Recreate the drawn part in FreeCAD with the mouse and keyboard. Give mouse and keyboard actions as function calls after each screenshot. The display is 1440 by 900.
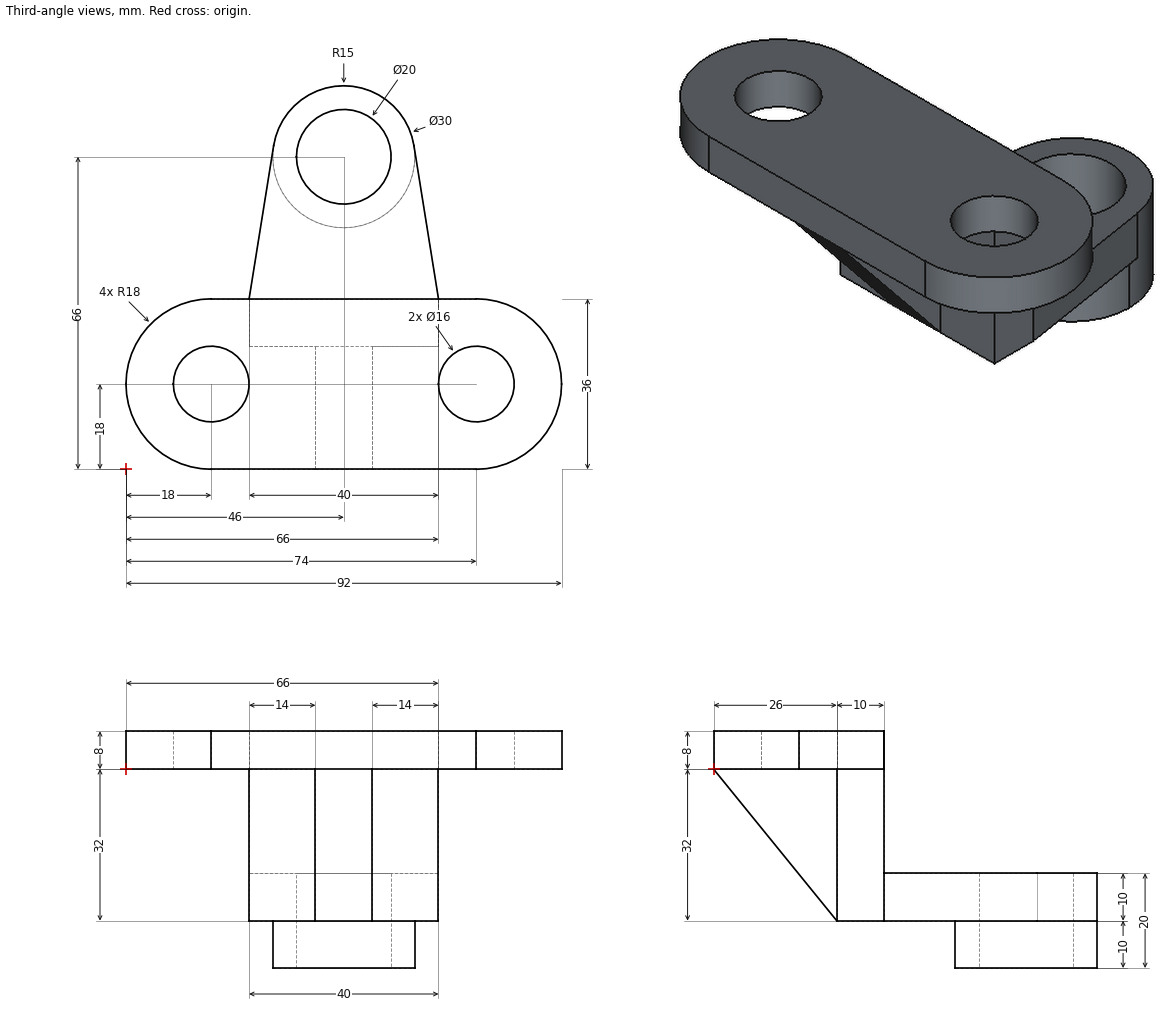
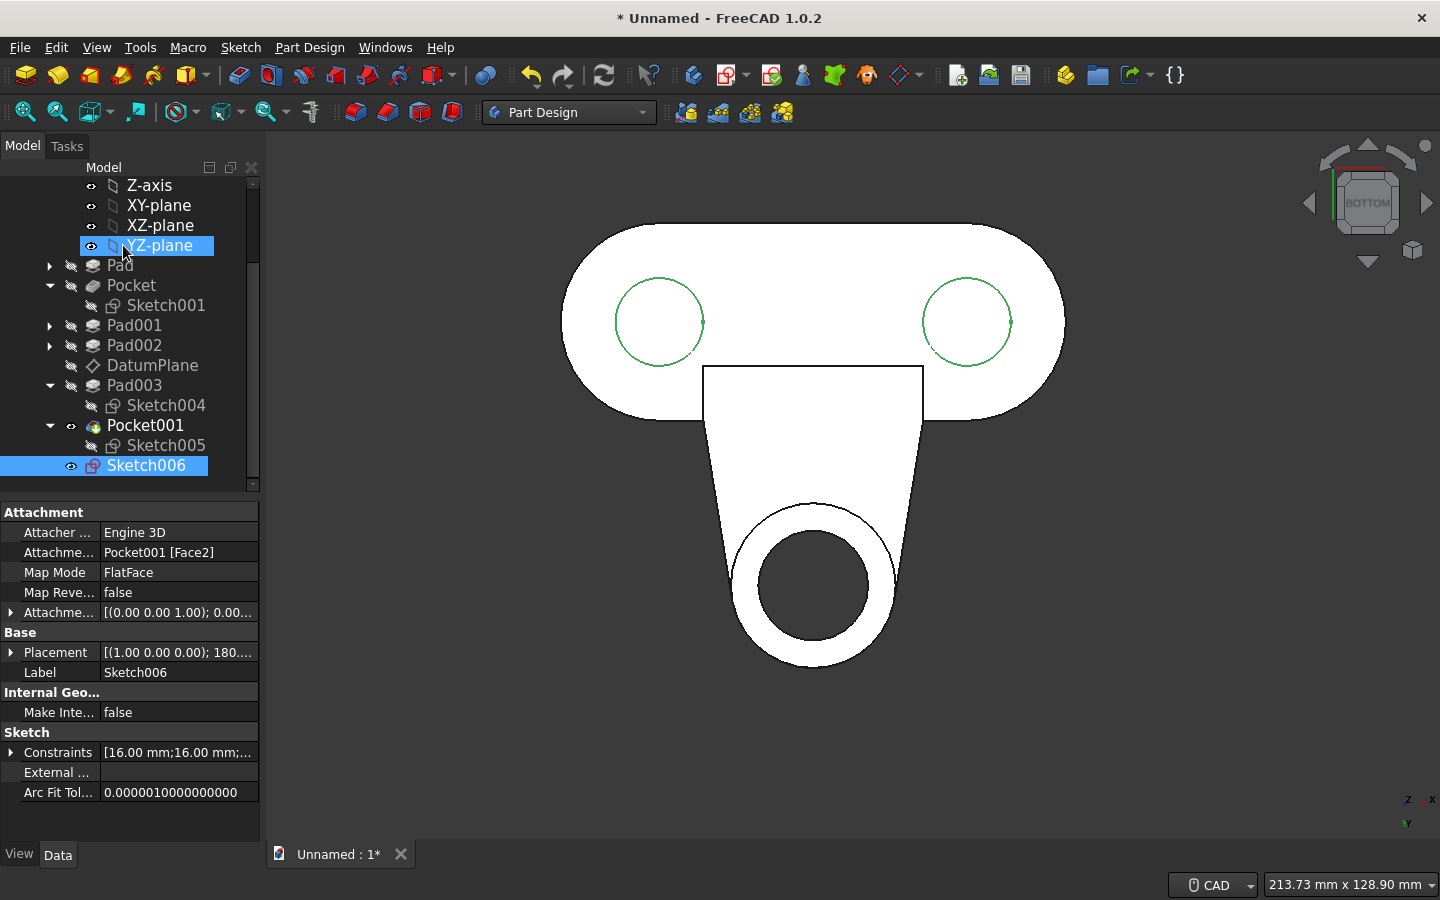
click(240, 76)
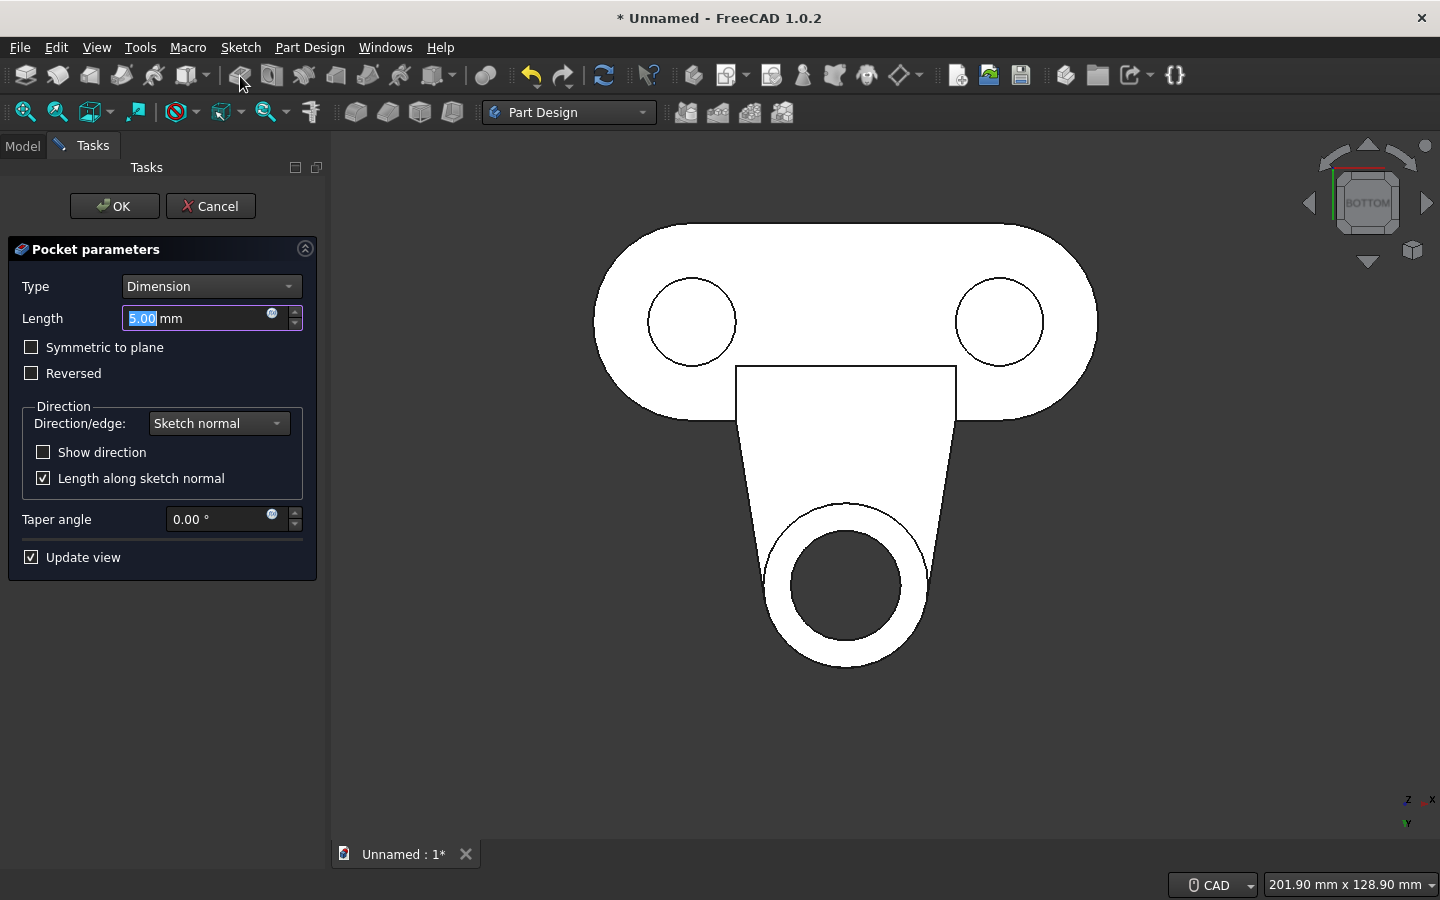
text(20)
key(Tab)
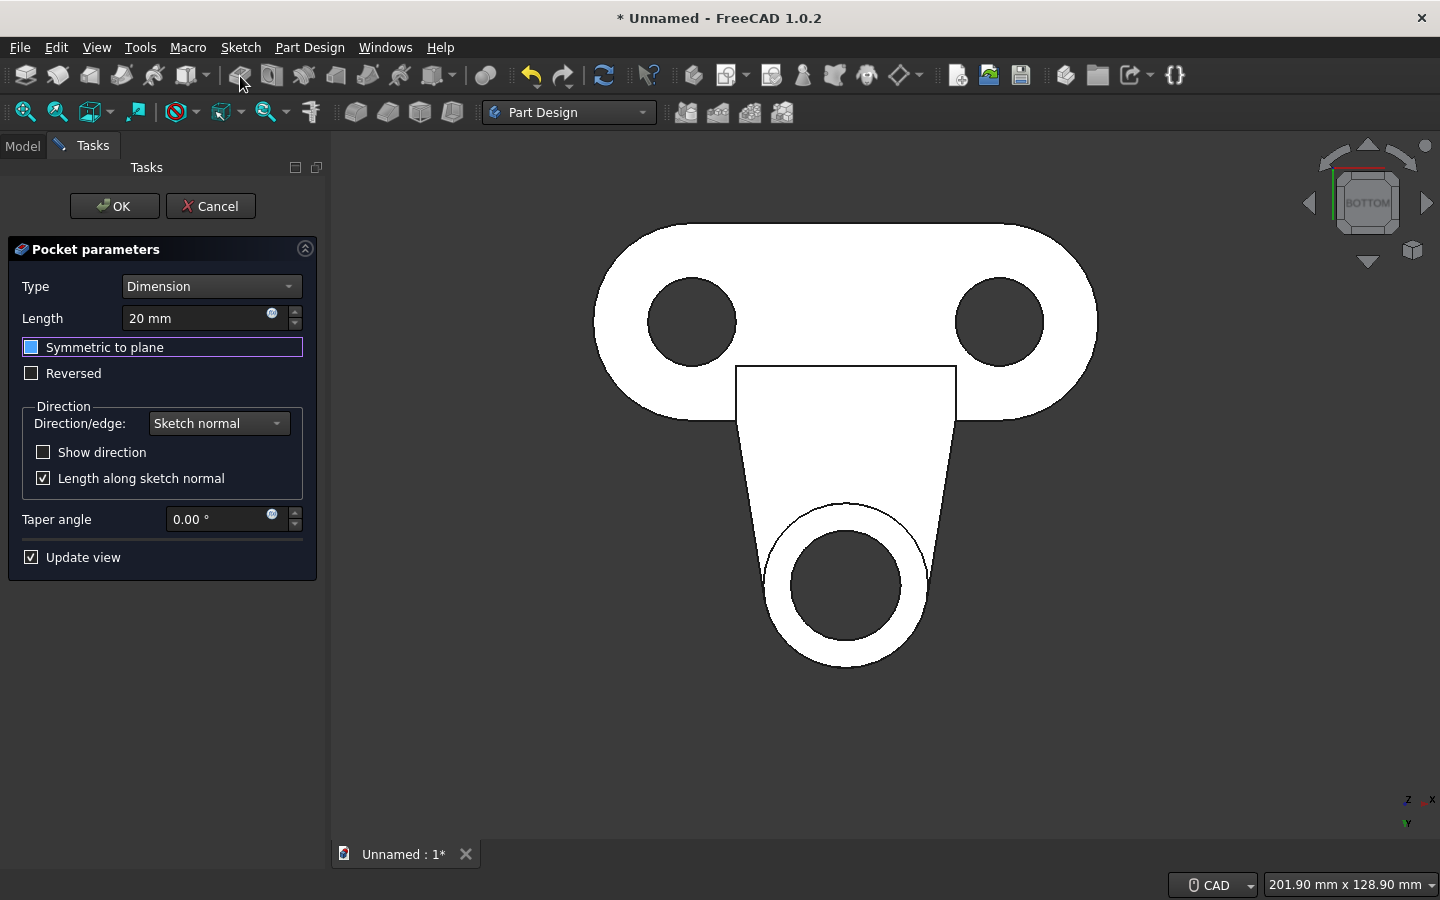
click(115, 206)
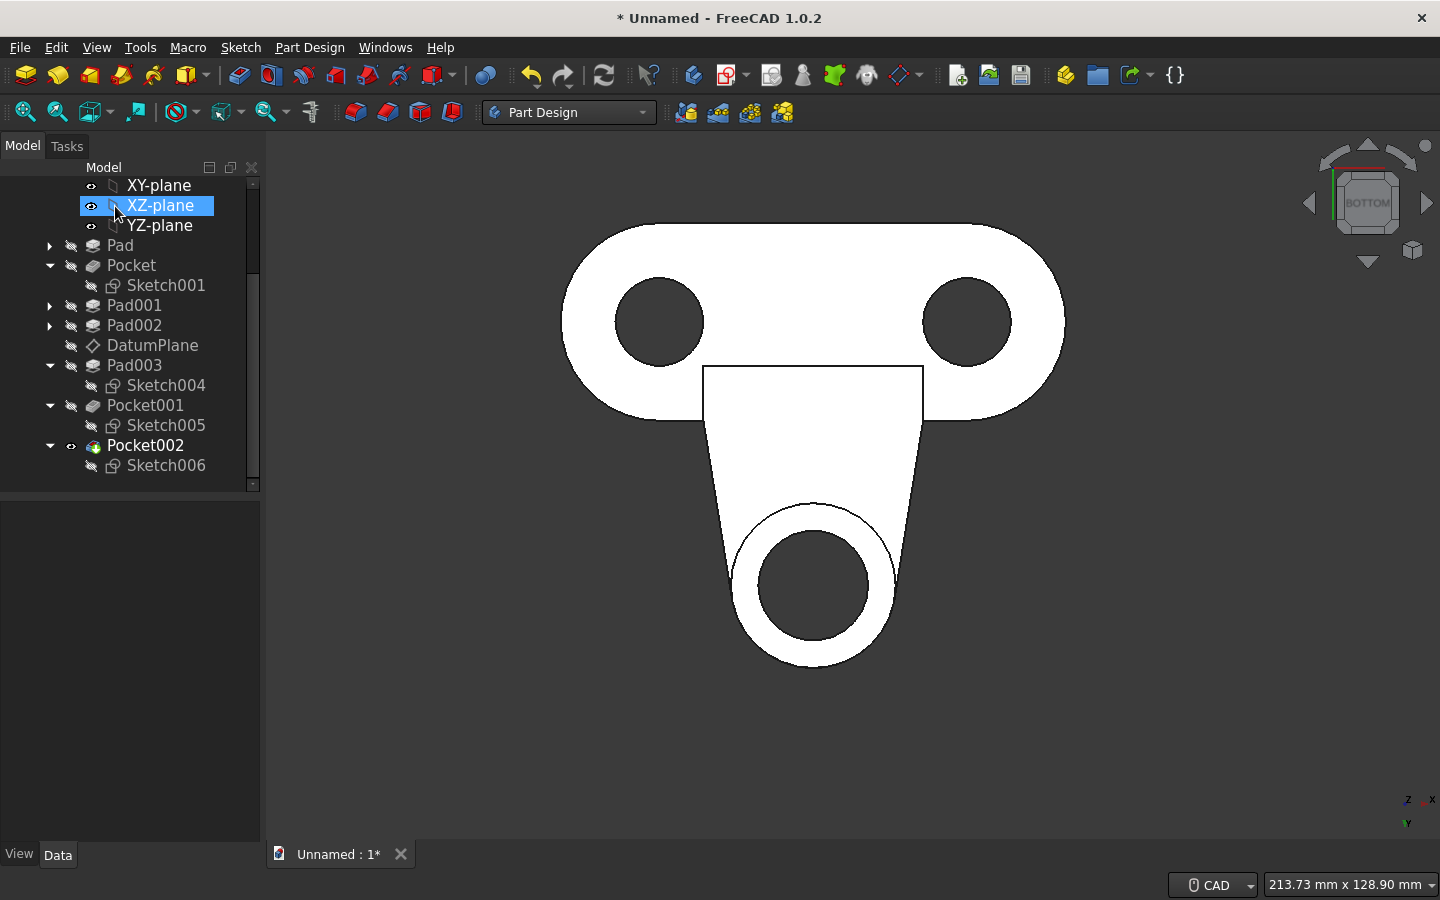
key(6)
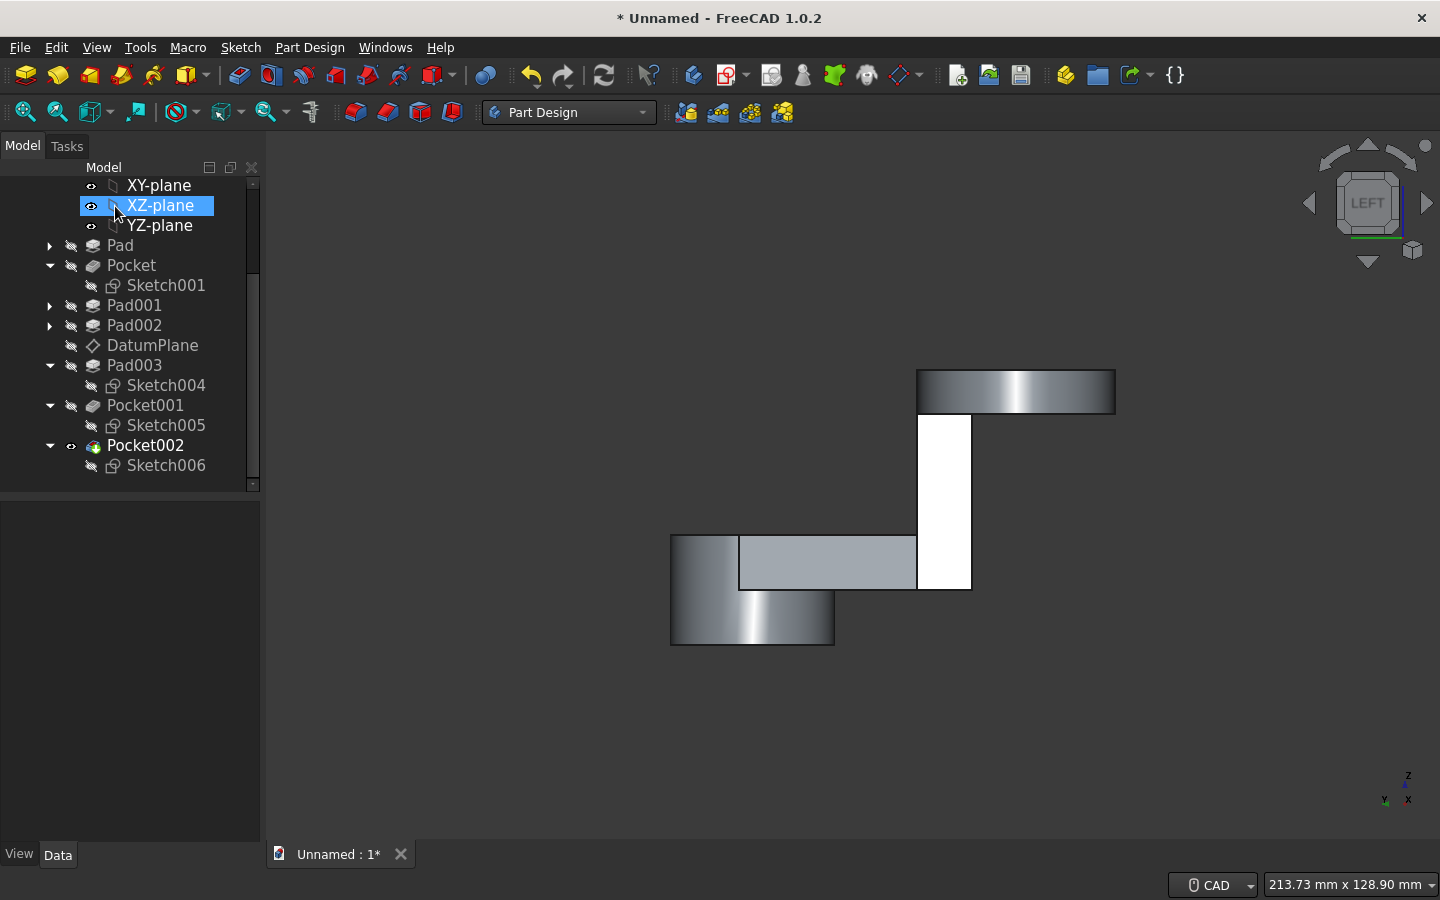
click(26, 112)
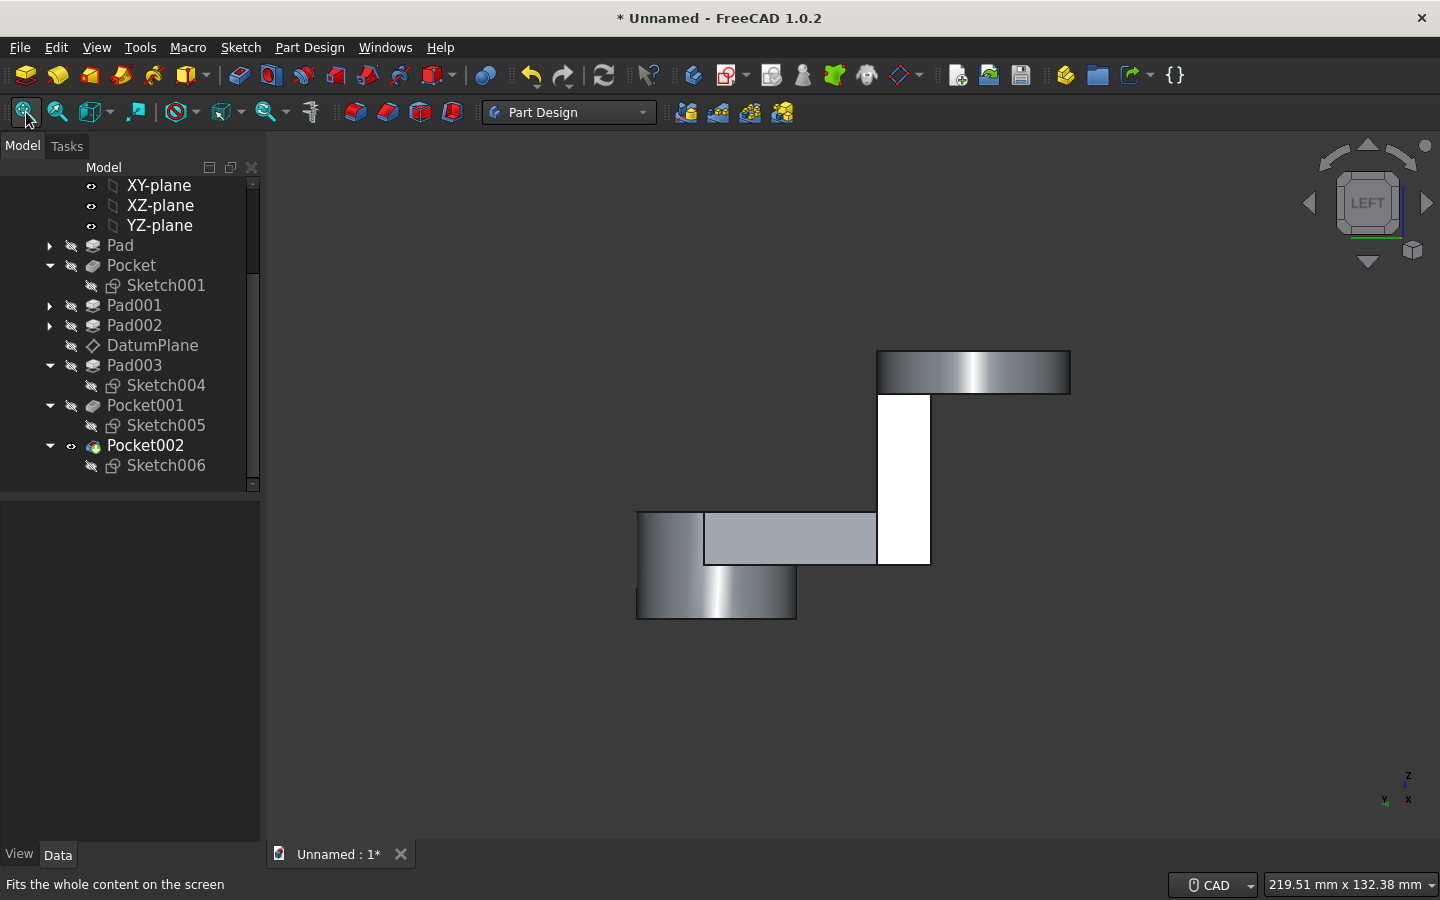
click(904, 430)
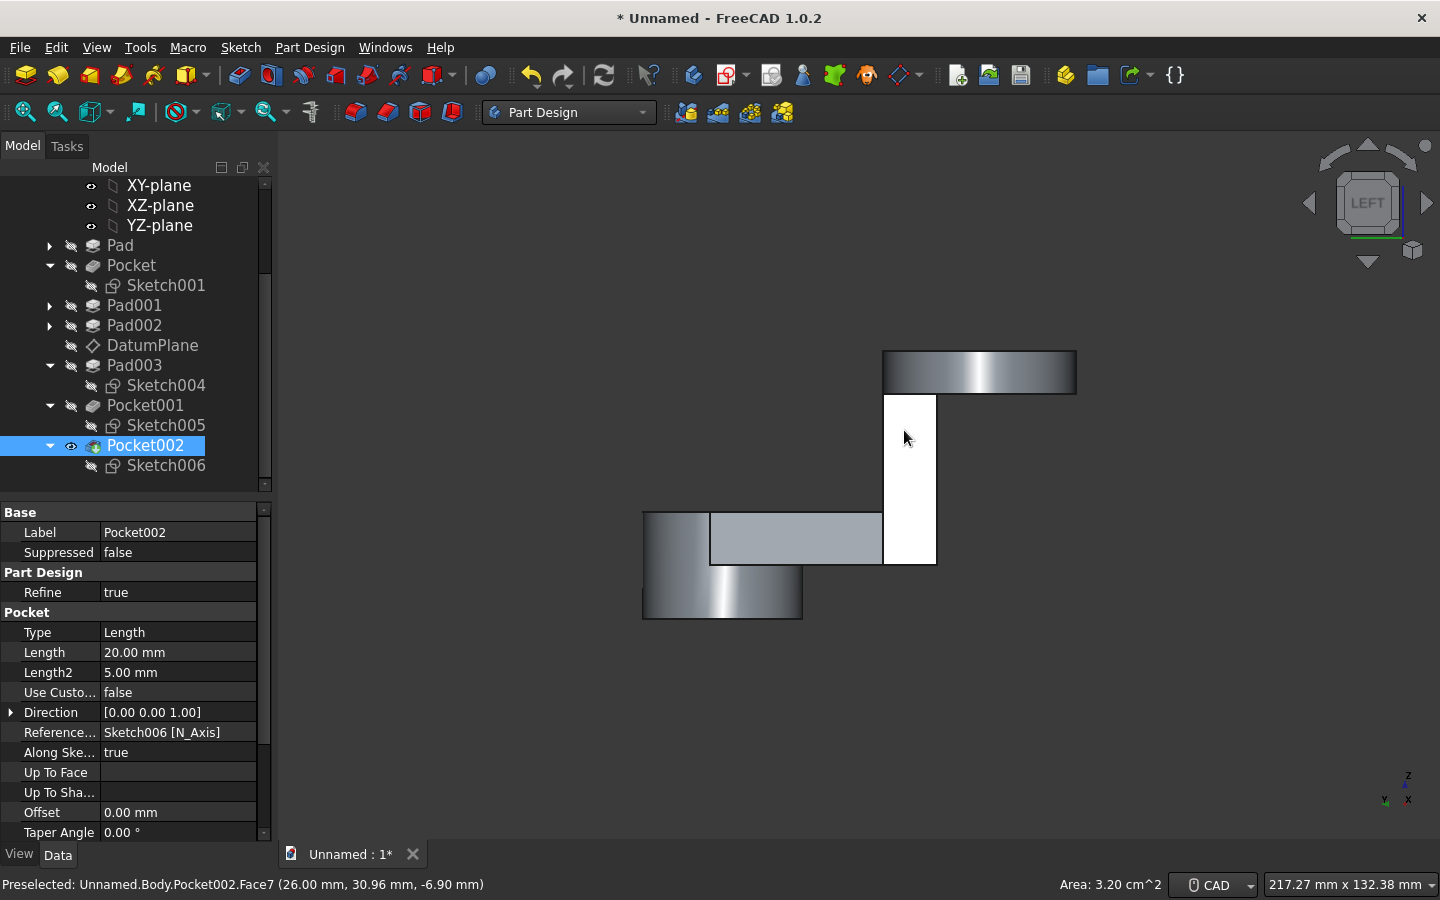
click(726, 76)